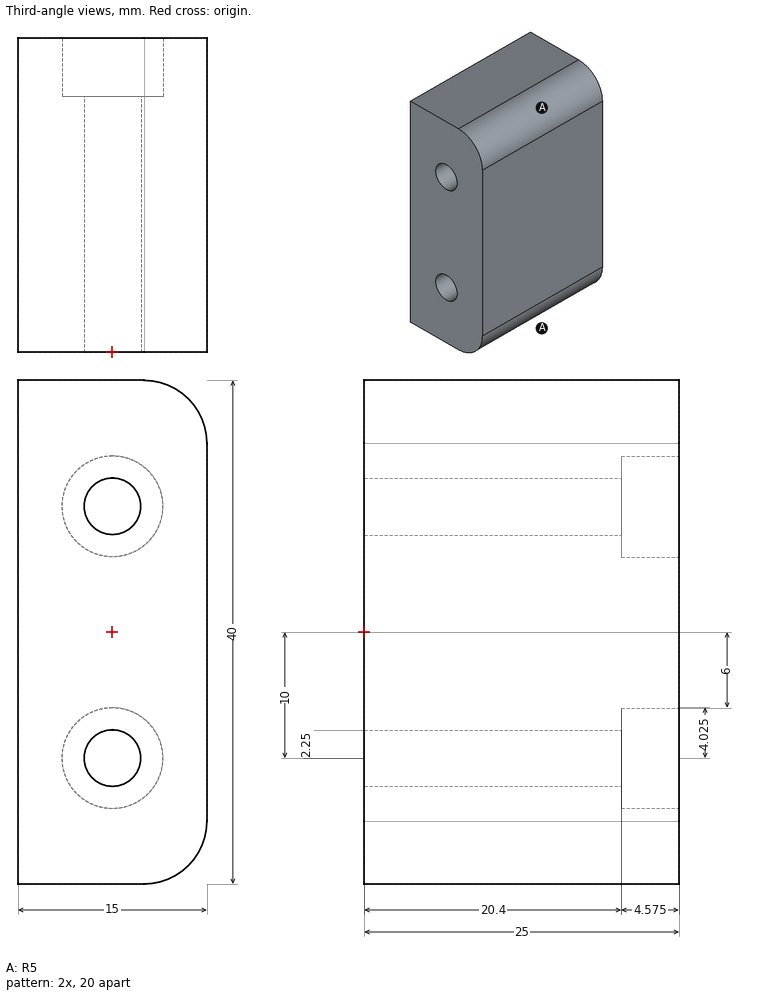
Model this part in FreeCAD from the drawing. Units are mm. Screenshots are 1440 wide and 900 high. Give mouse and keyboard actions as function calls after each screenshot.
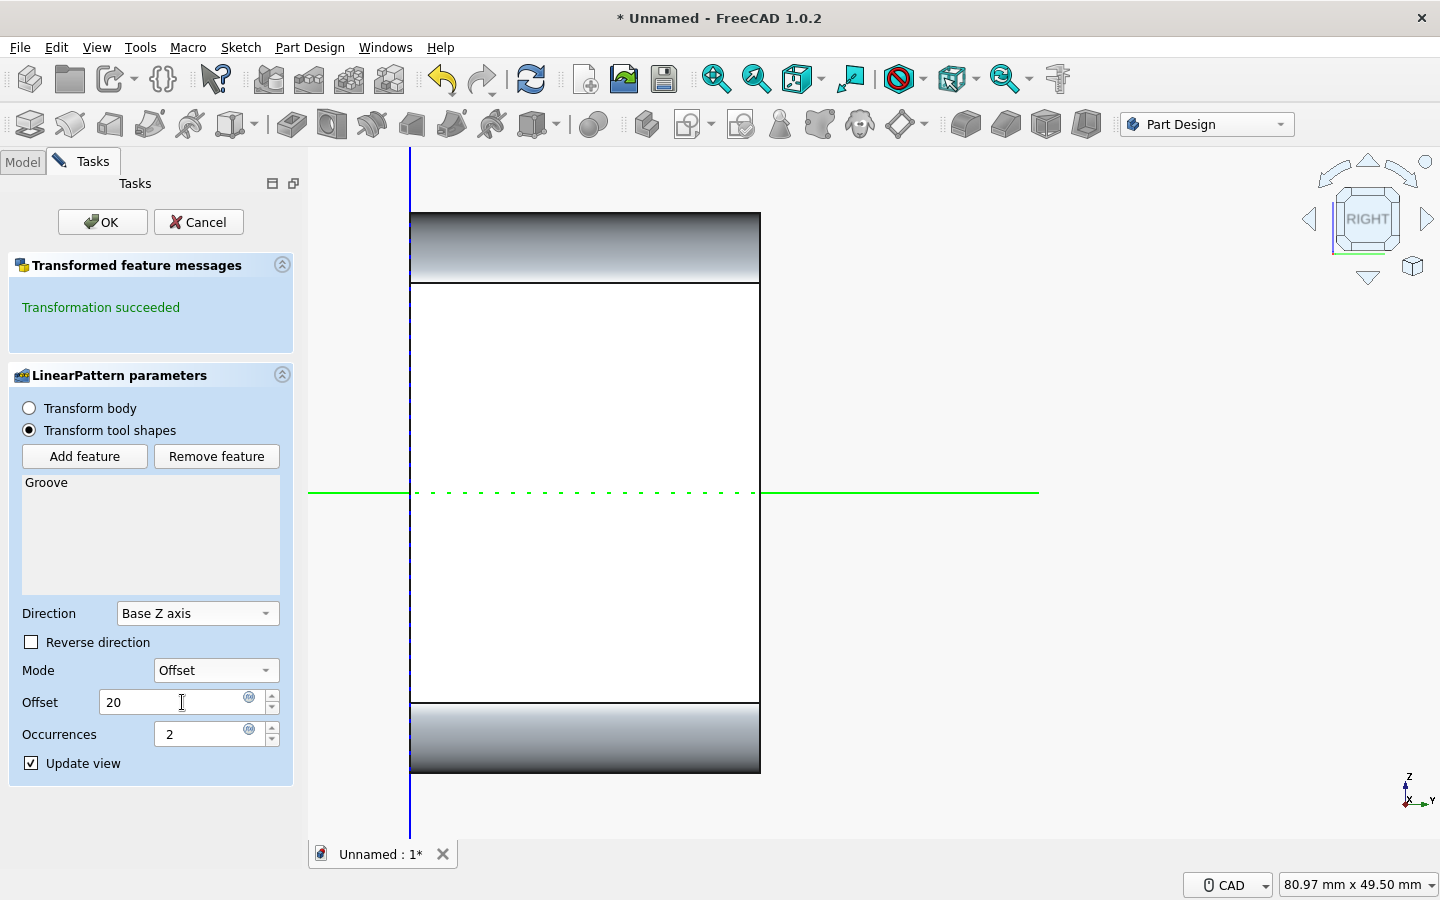
triple_click(209, 734)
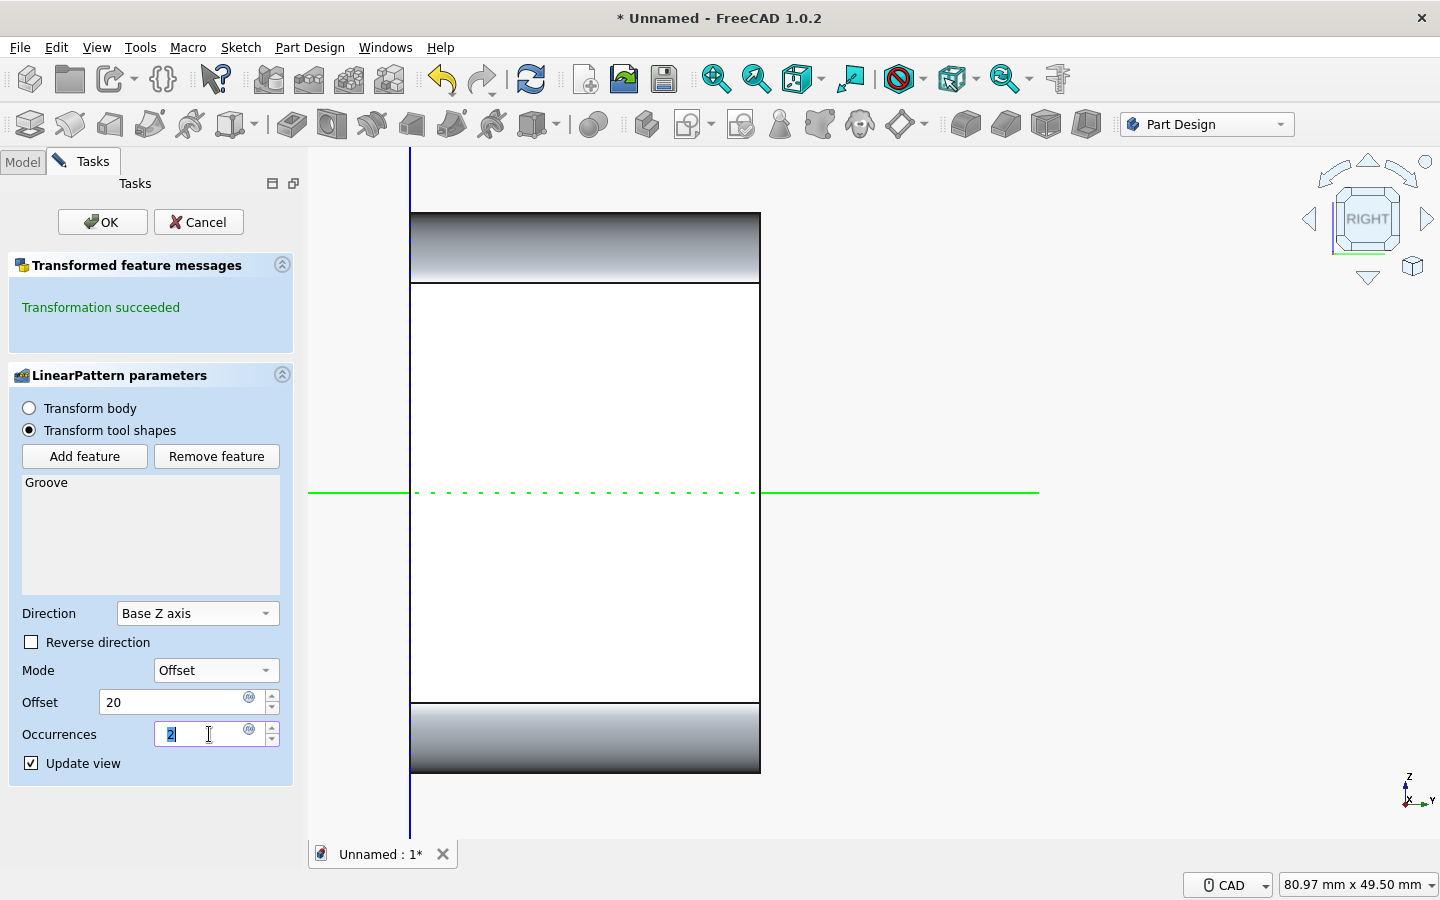
text(2)
key(Tab)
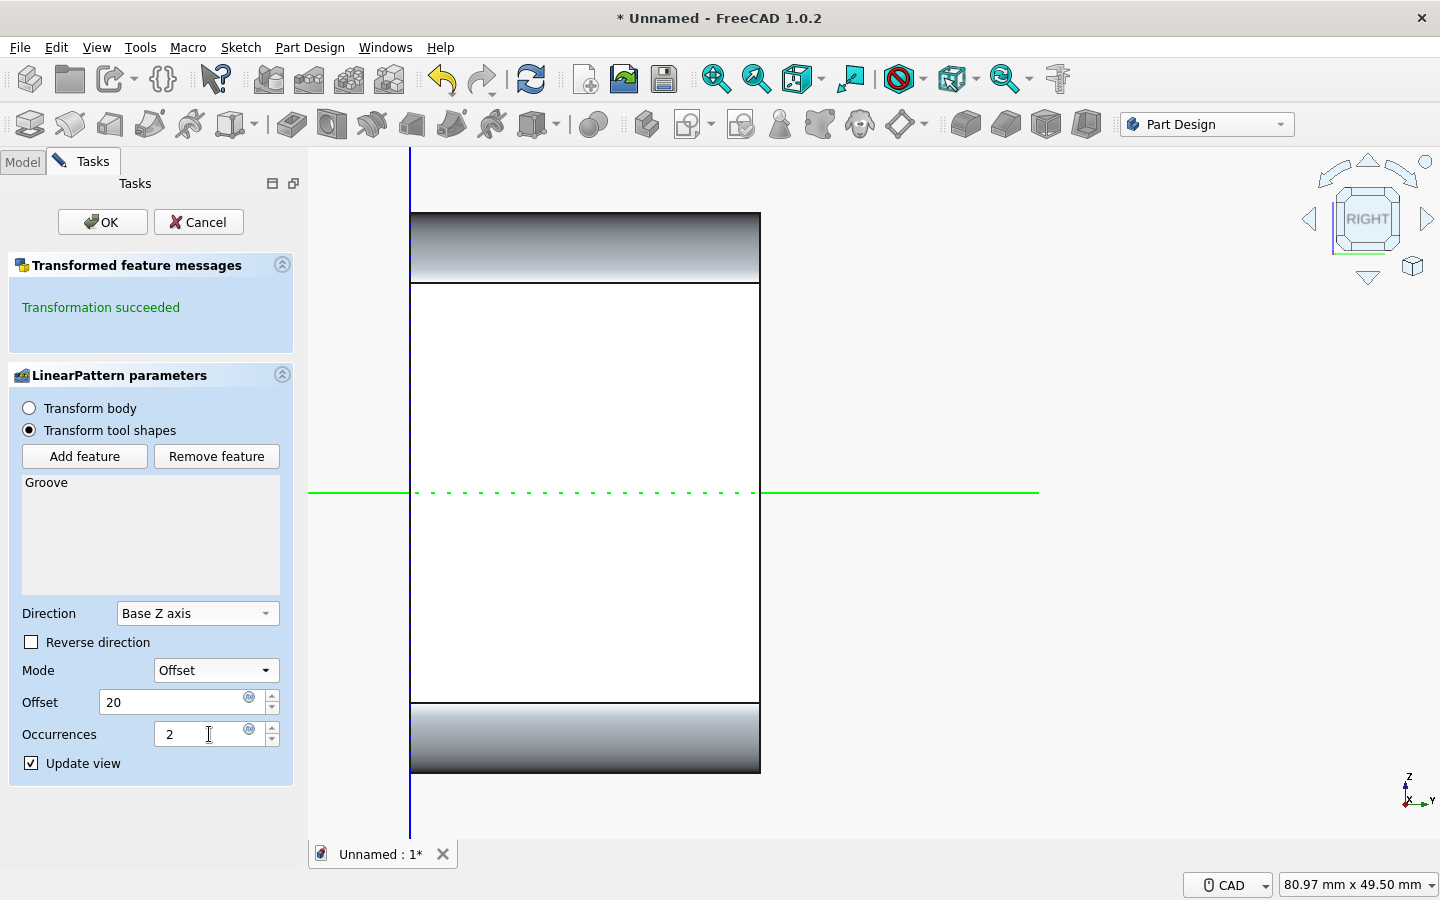
click(103, 222)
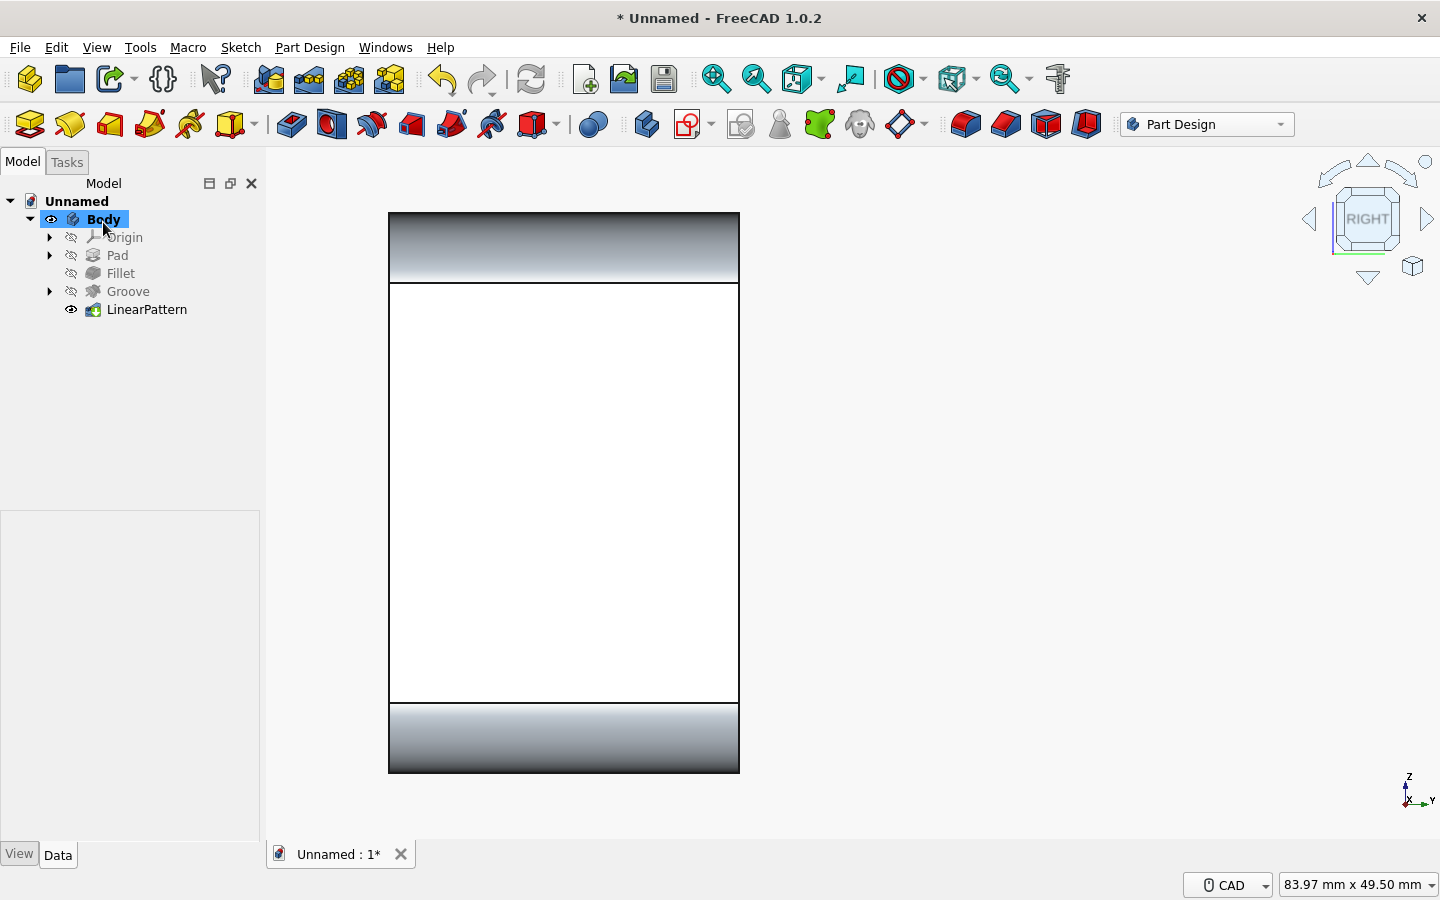
key(0)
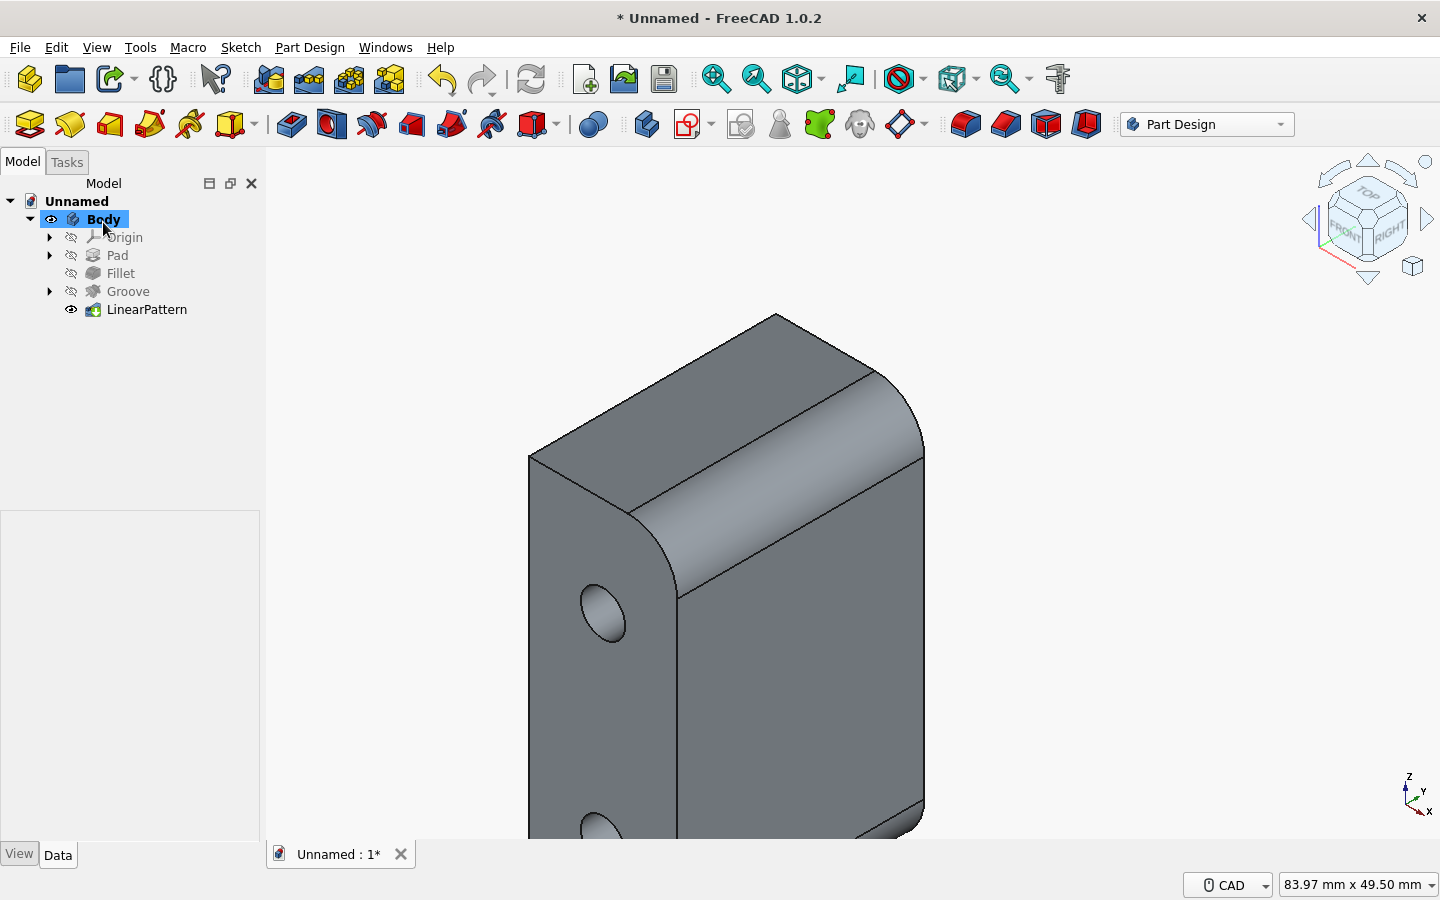
click(718, 80)